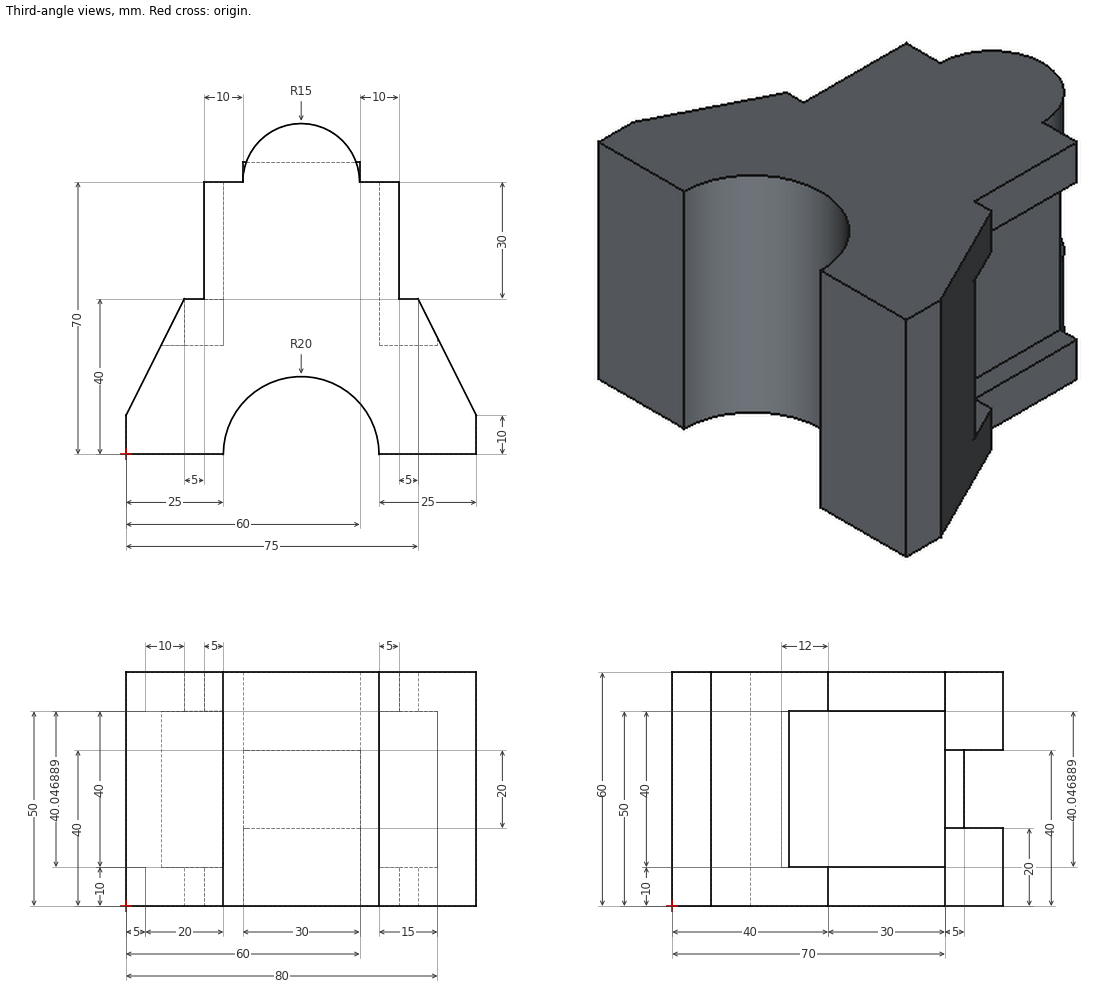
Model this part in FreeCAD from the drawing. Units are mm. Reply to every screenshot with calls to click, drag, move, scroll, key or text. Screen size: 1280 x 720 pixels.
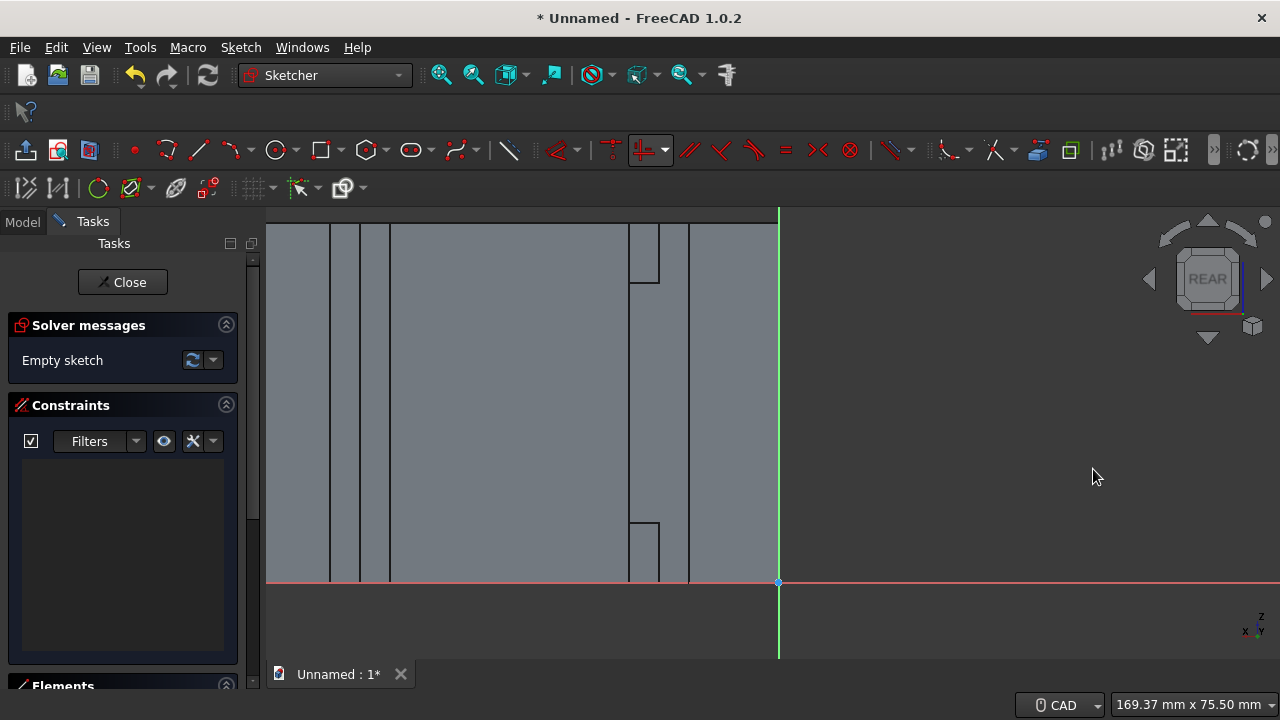
key(g)
key(m)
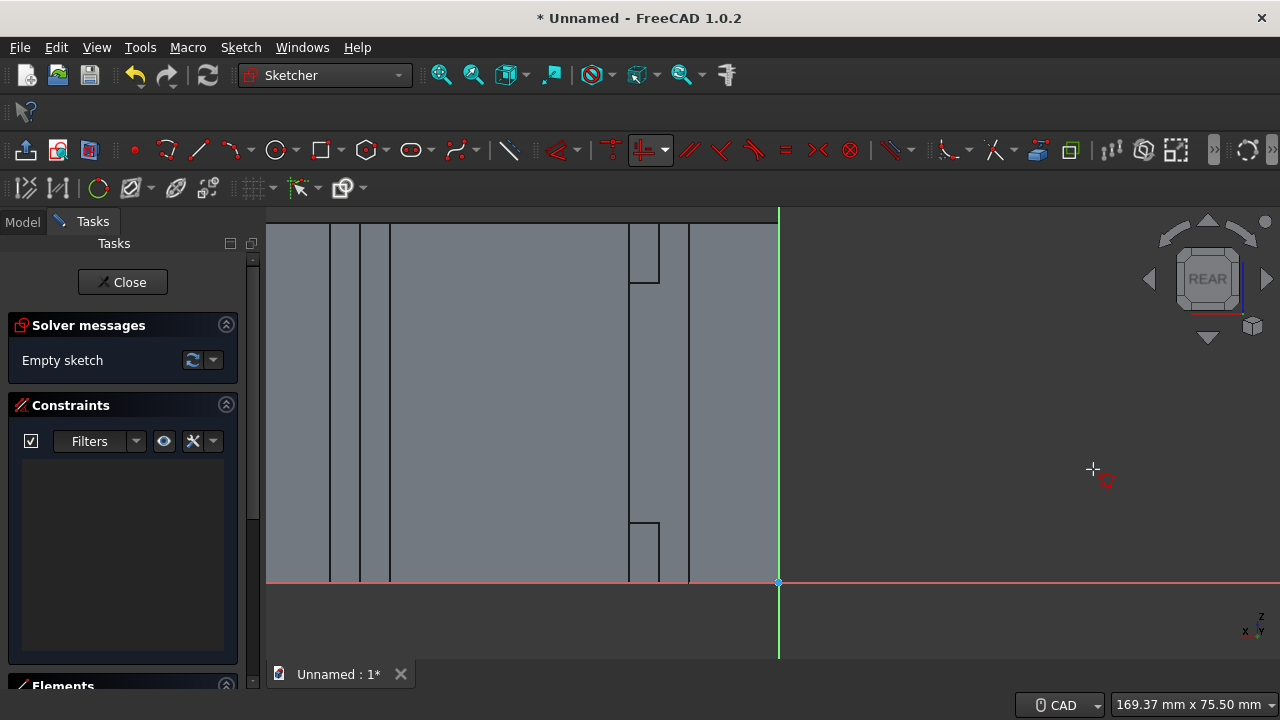
click(749, 523)
click(749, 283)
click(689, 283)
click(629, 279)
click(629, 523)
click(749, 524)
key(Escape)
key(Escape)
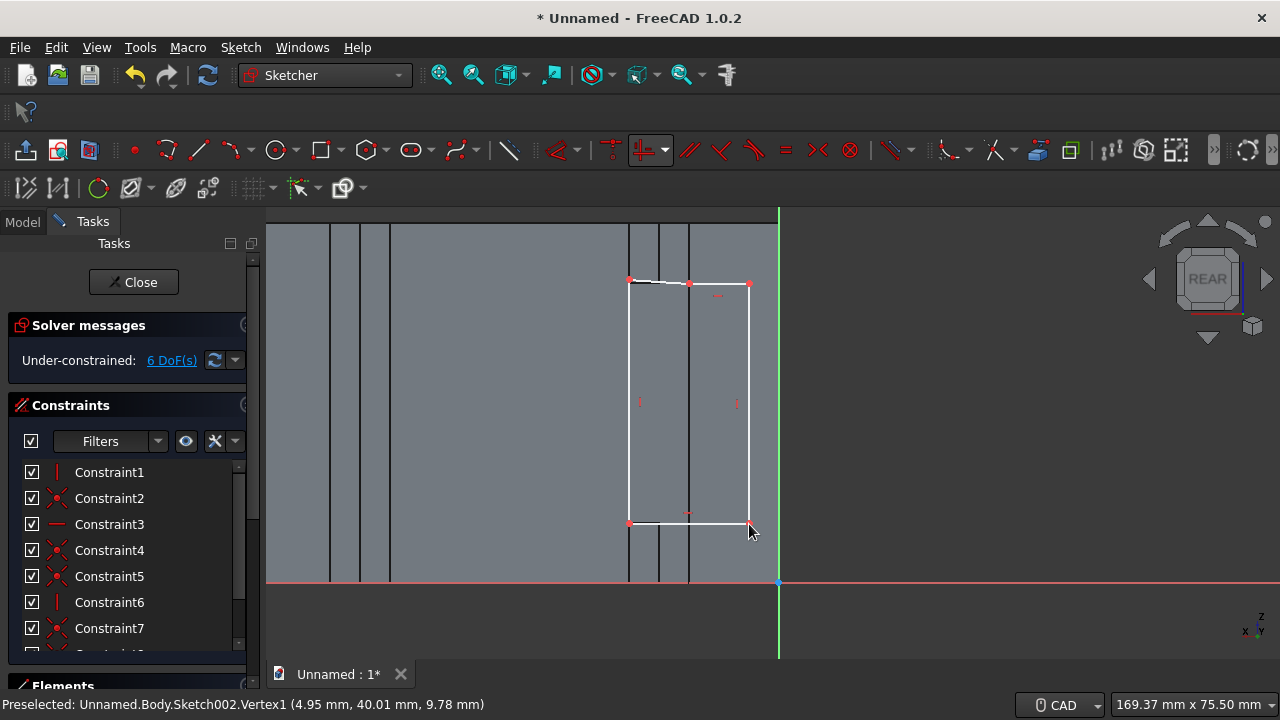
key(d)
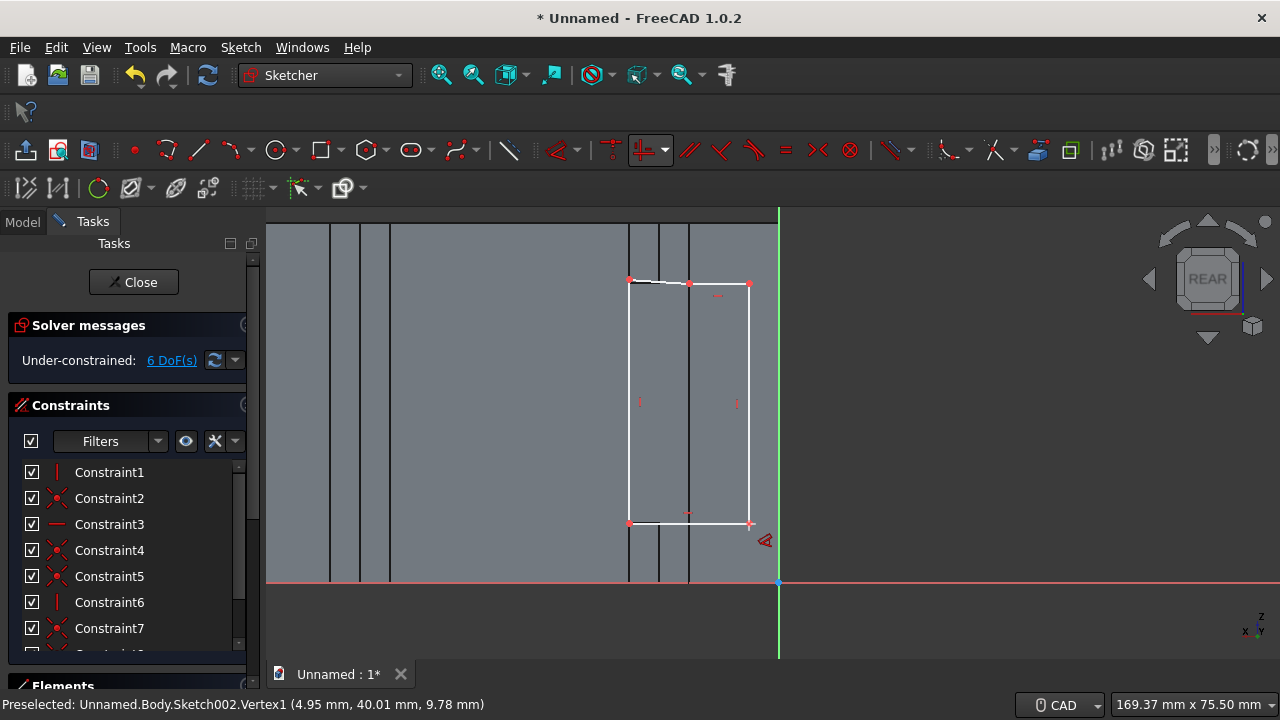
click(749, 452)
click(715, 404)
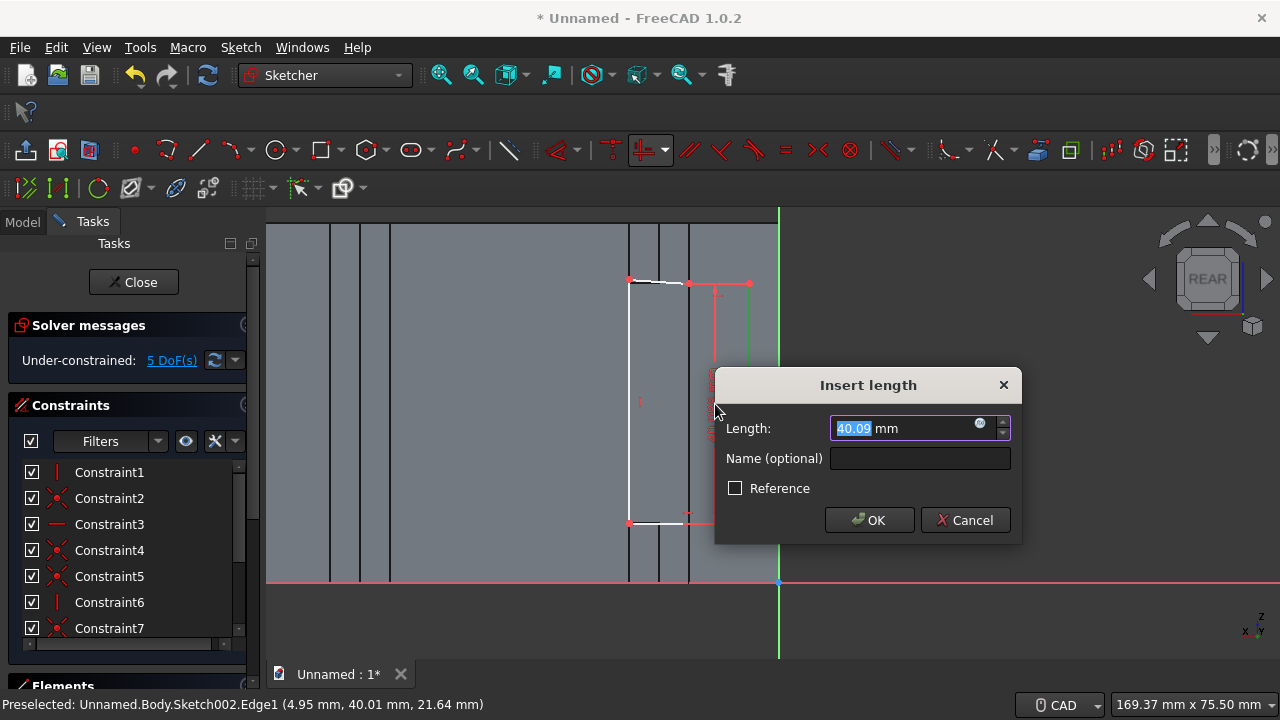
text(40)
key(Return)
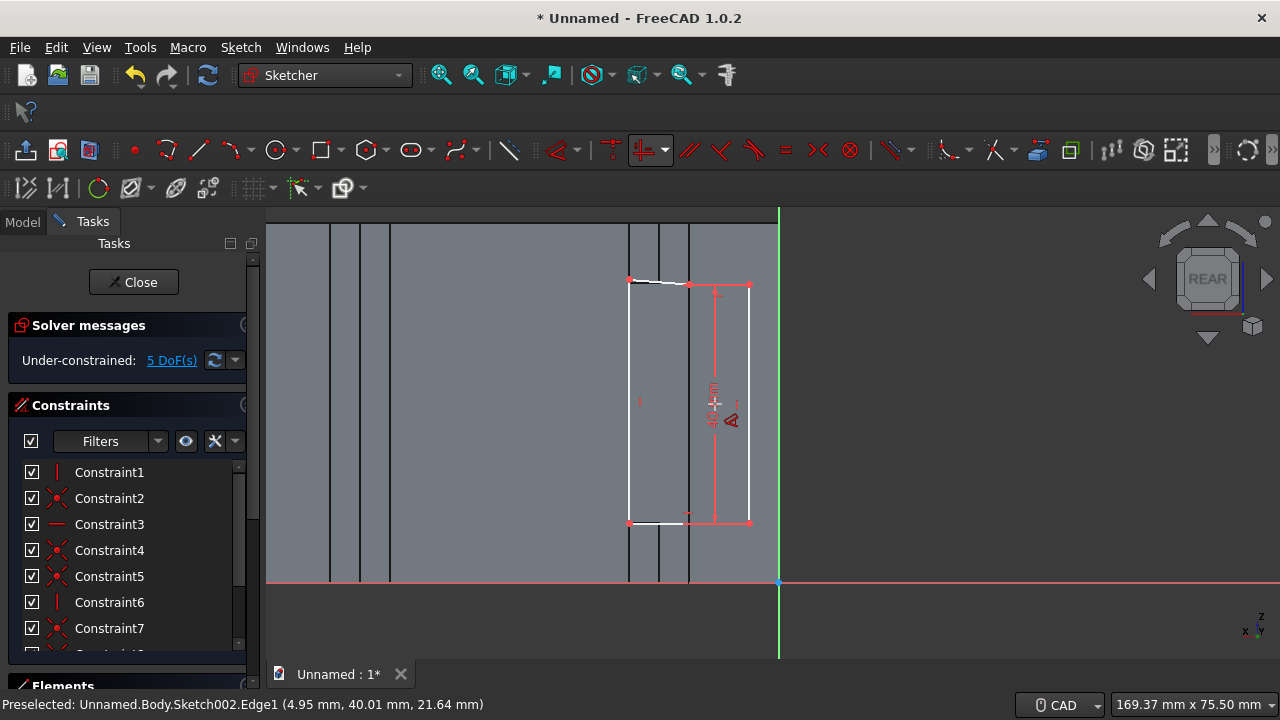
click(731, 285)
click(719, 251)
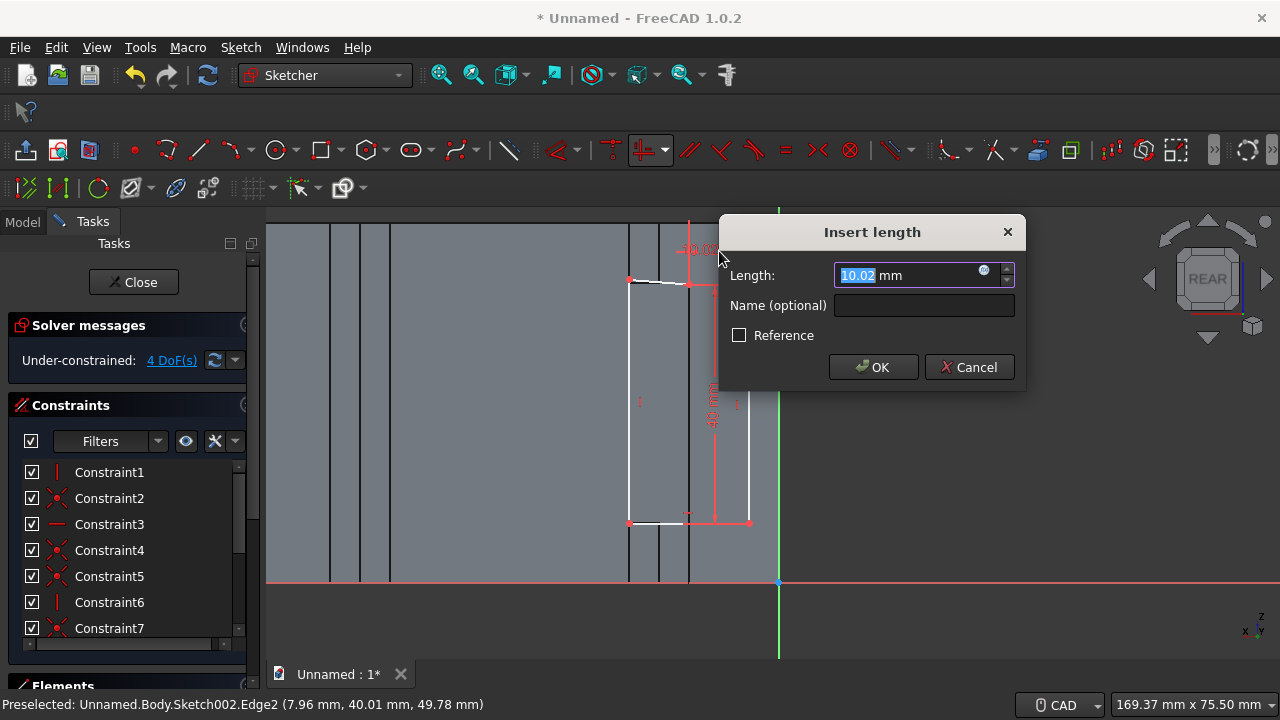
text(10)
key(Return)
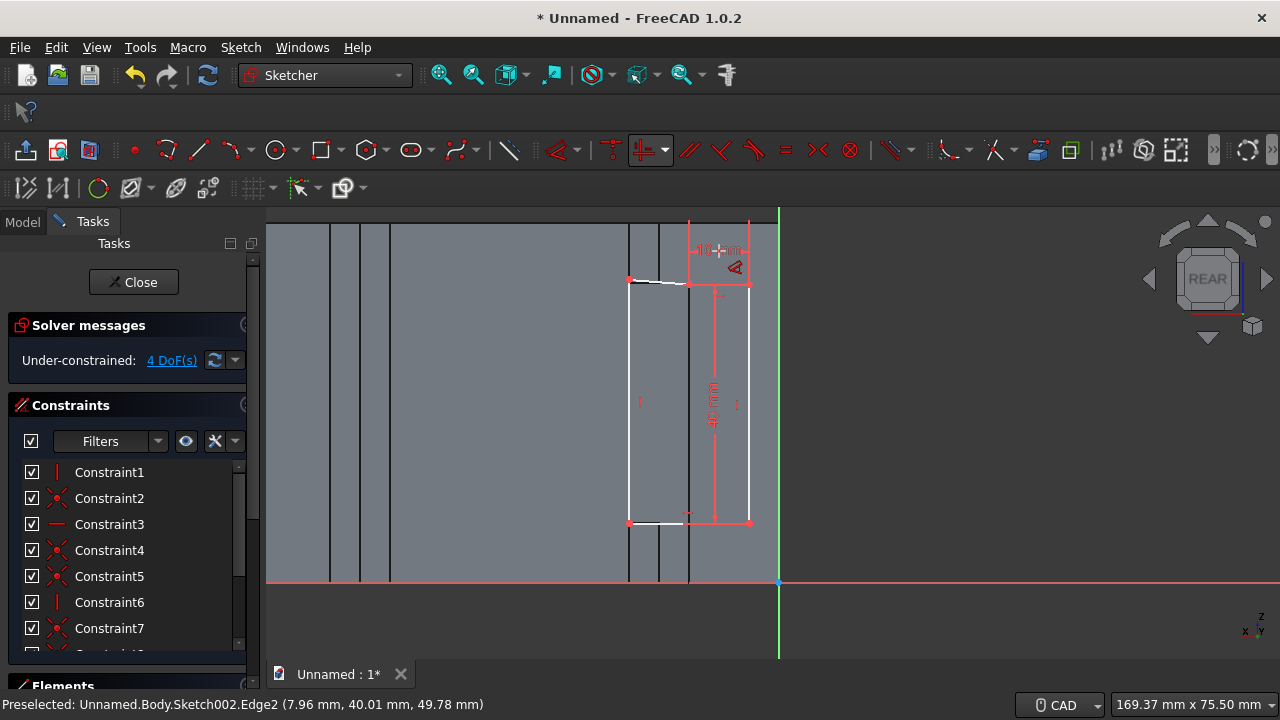
click(665, 524)
click(689, 558)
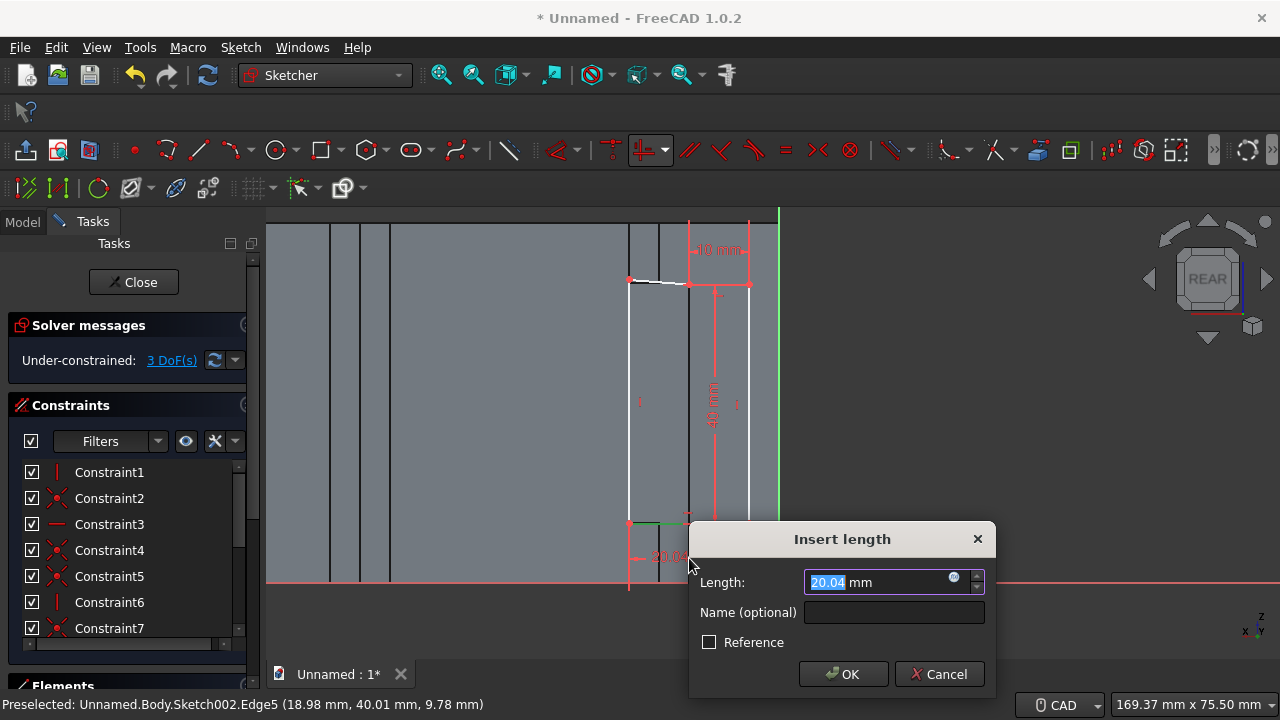
text(20)
key(Return)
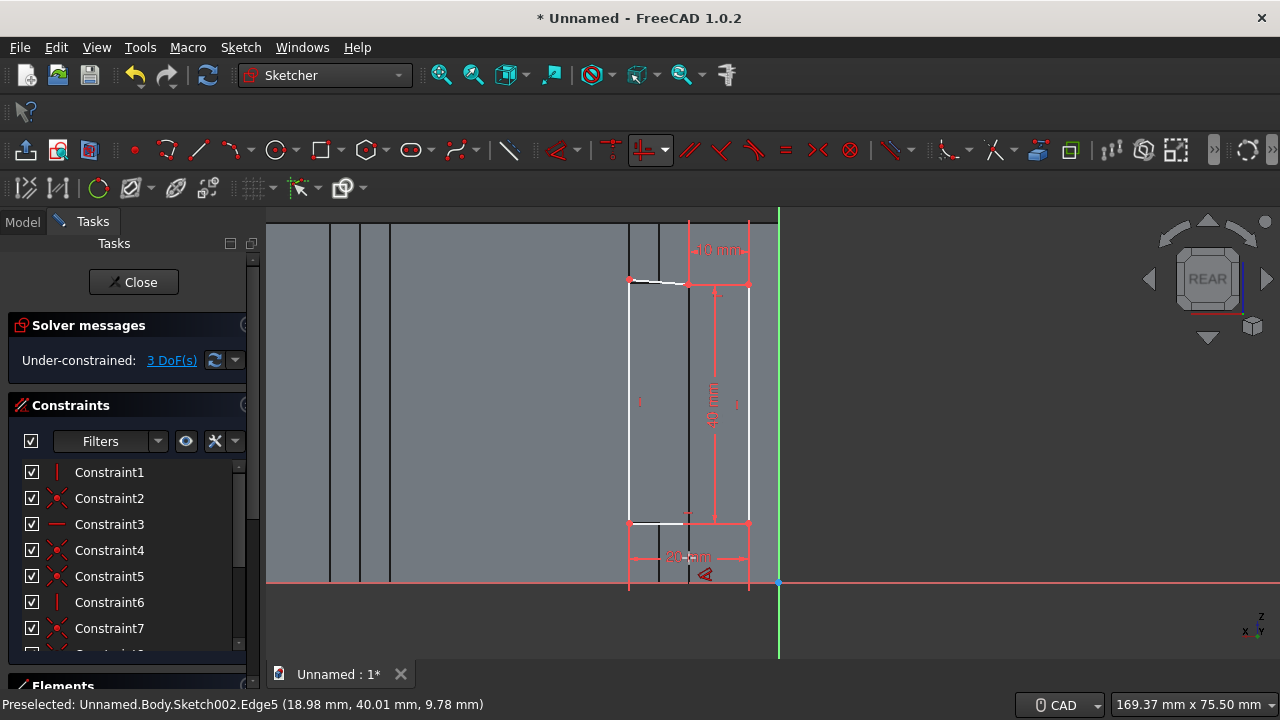
scroll(749, 524, up, 2)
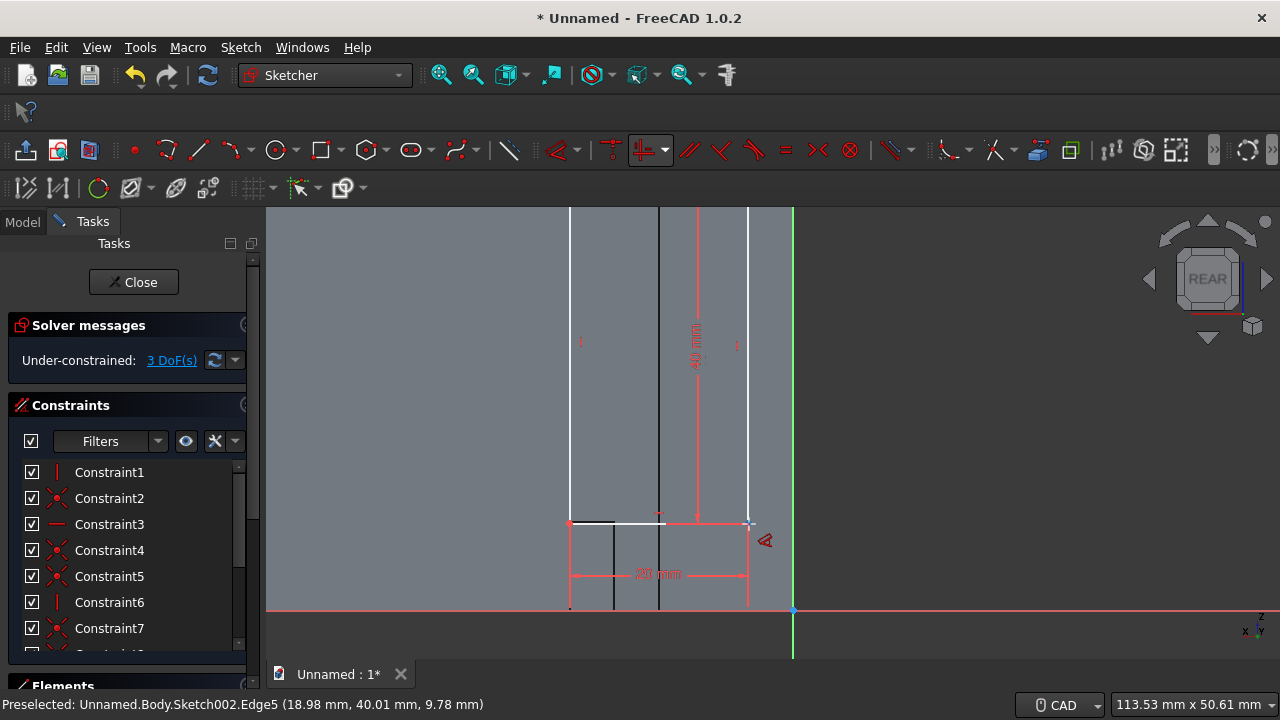
click(748, 524)
click(771, 490)